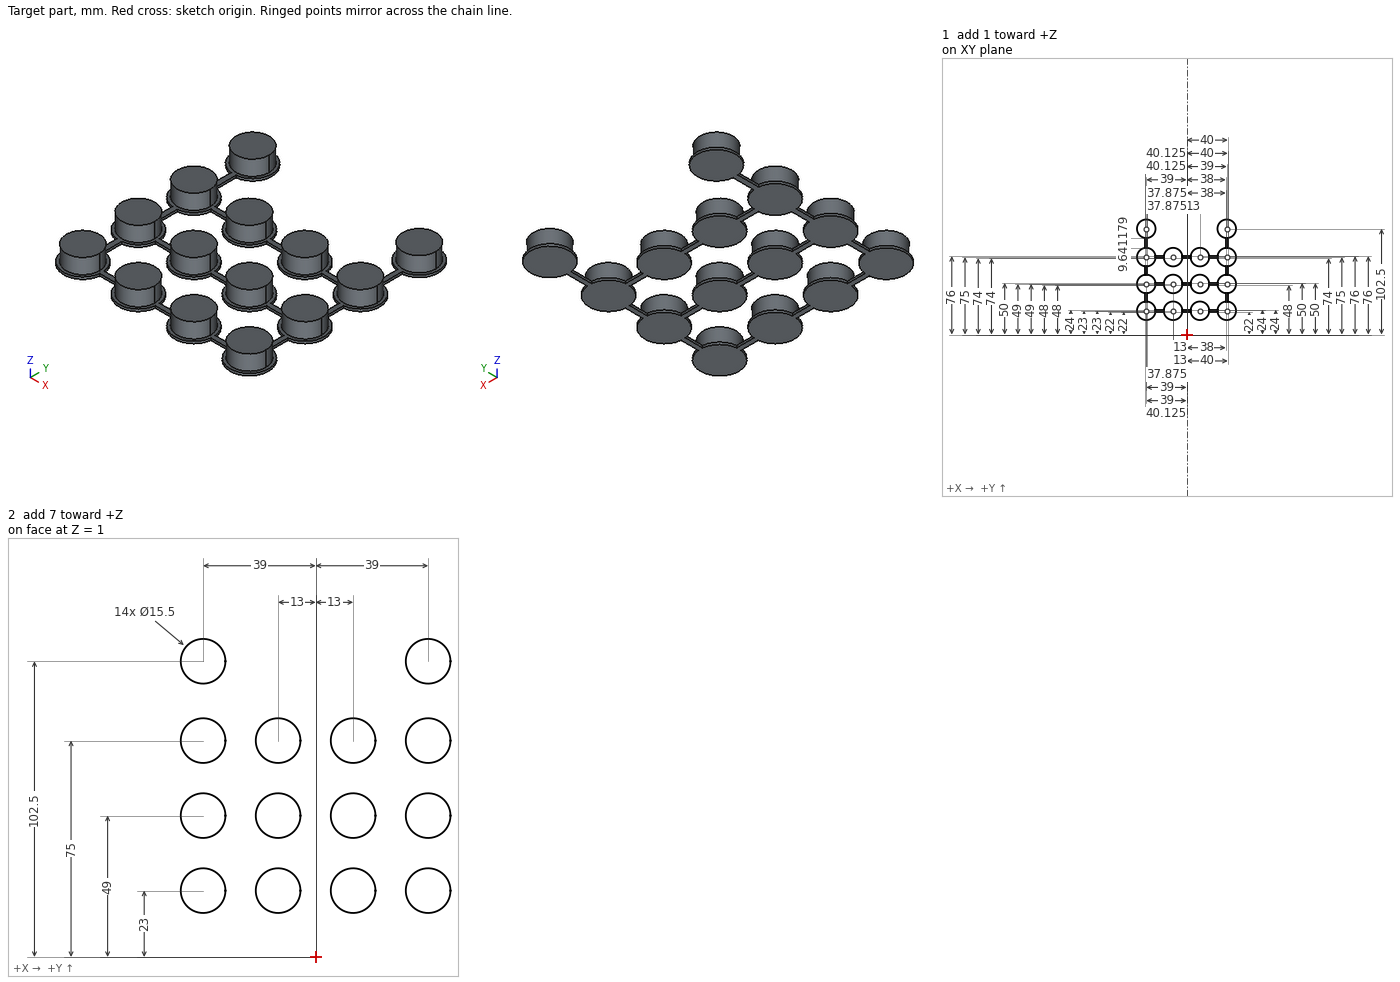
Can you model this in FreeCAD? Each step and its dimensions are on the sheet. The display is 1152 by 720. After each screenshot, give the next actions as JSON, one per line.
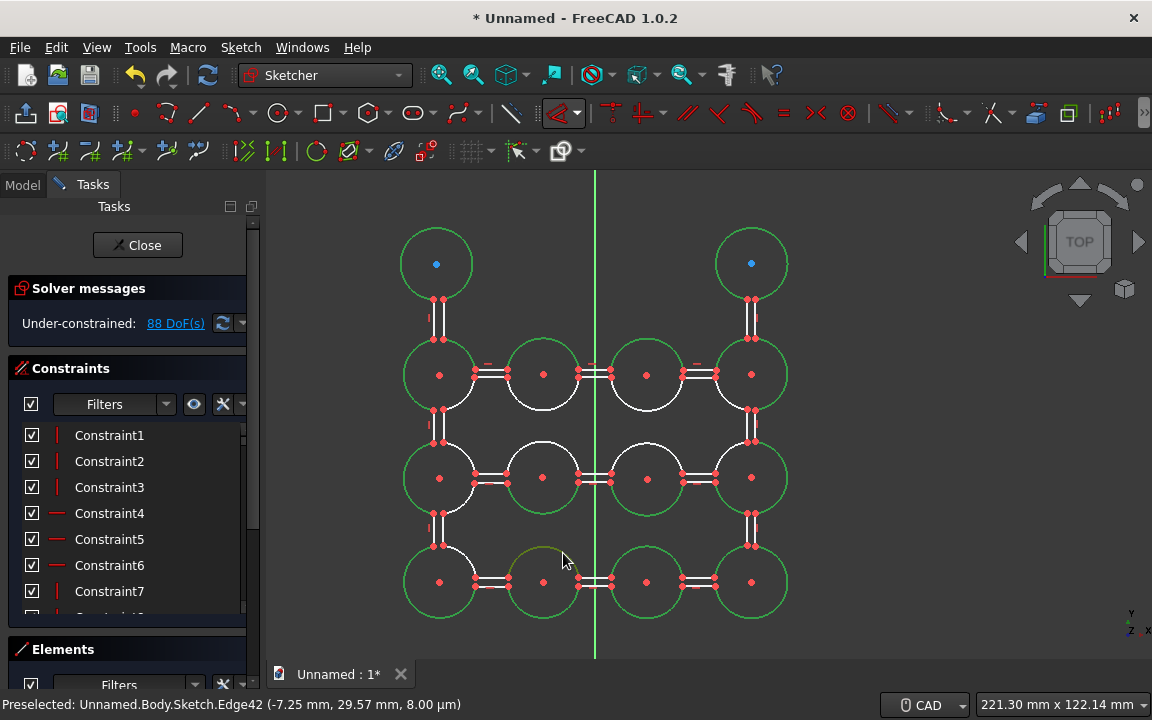
{"action": "left_click", "coordinate": [471, 564]}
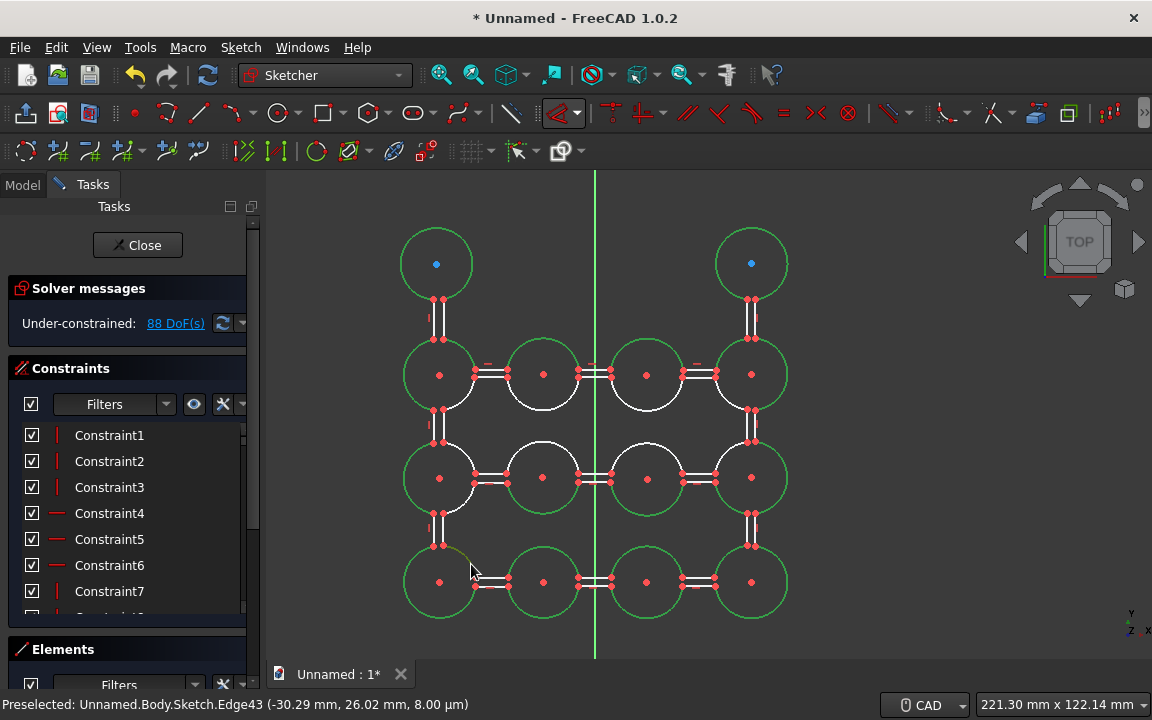
{"action": "left_click", "coordinate": [457, 509]}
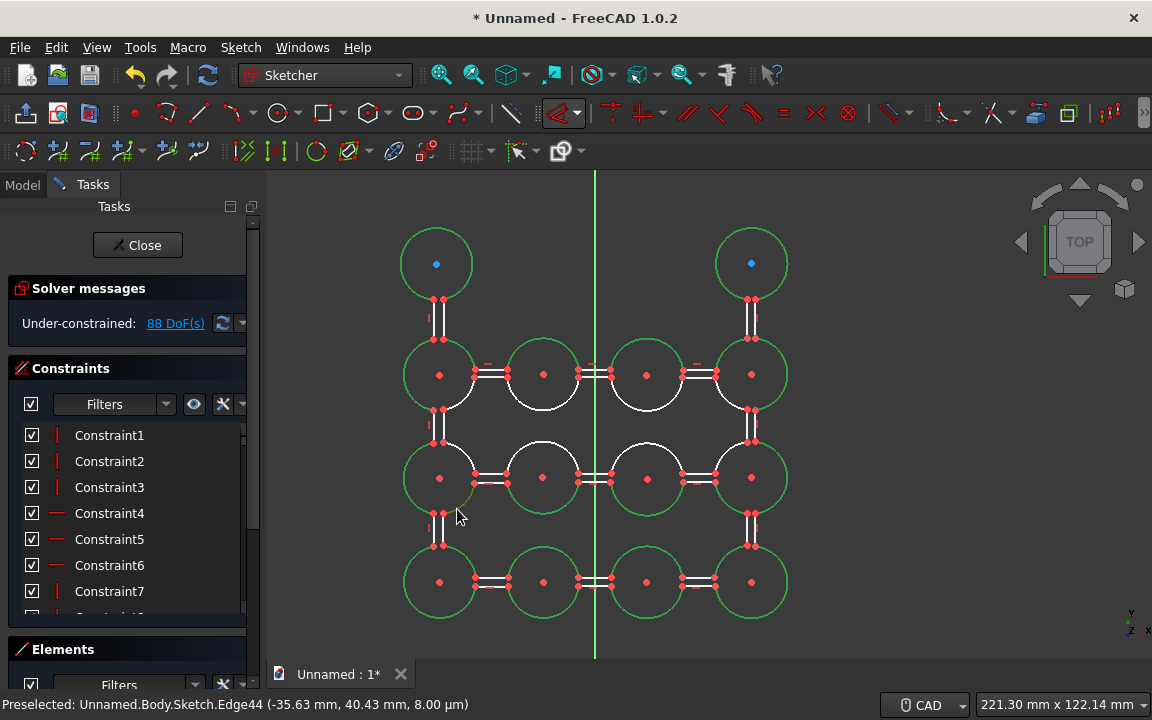
{"action": "left_click", "coordinate": [523, 404]}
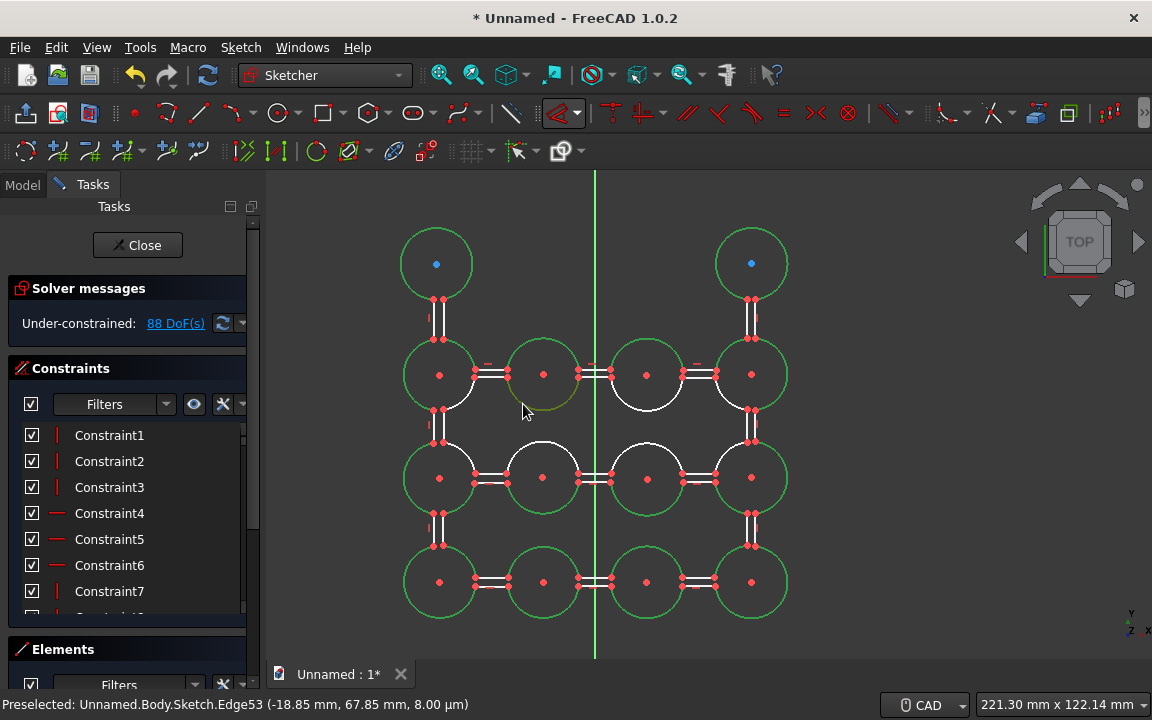
{"action": "left_click", "coordinate": [627, 405]}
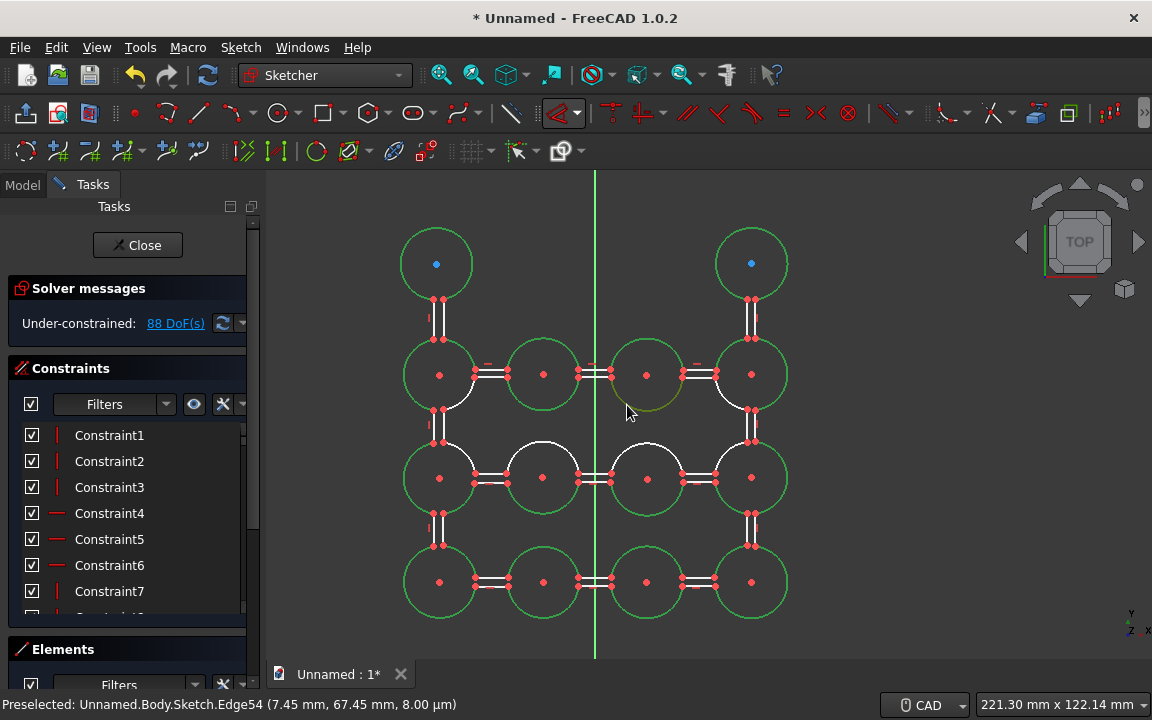
{"action": "left_click", "coordinate": [720, 392]}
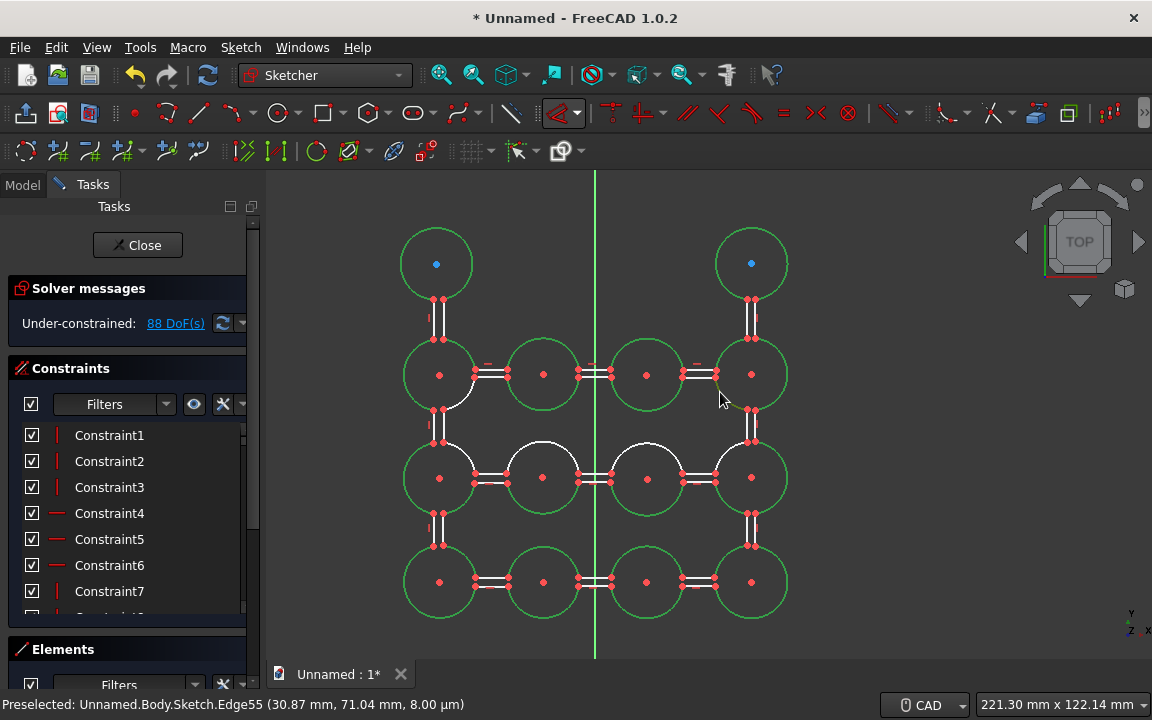
{"action": "left_click", "coordinate": [734, 446]}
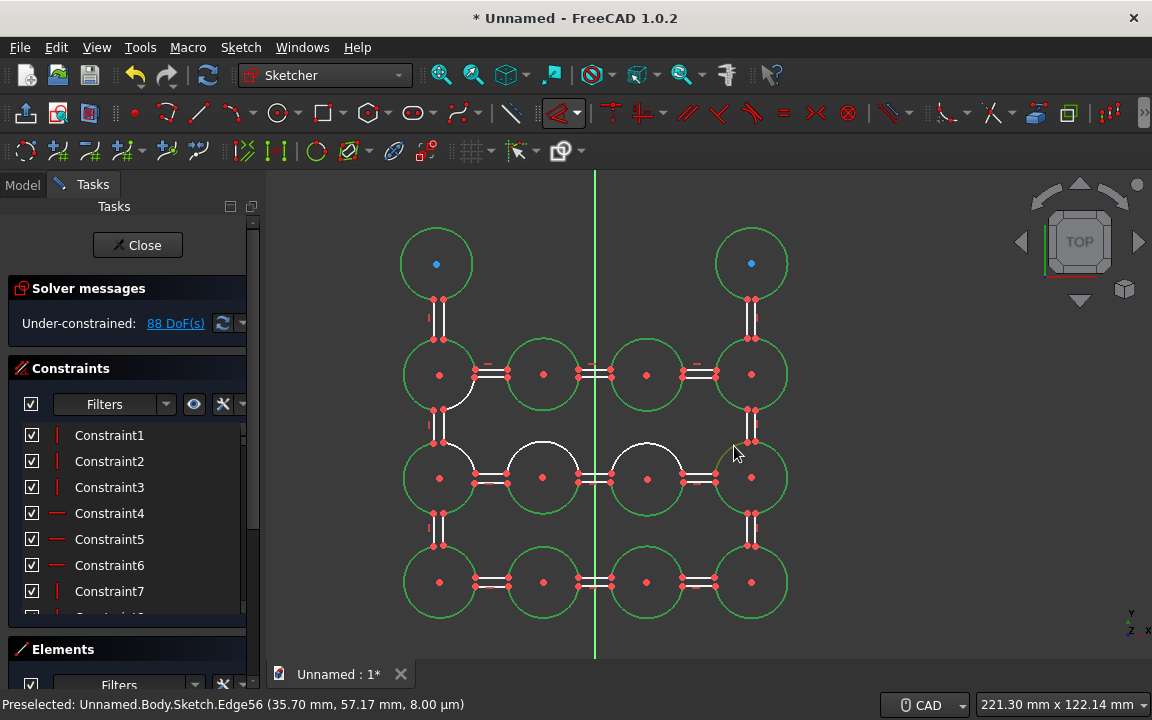
{"action": "left_click", "coordinate": [666, 449]}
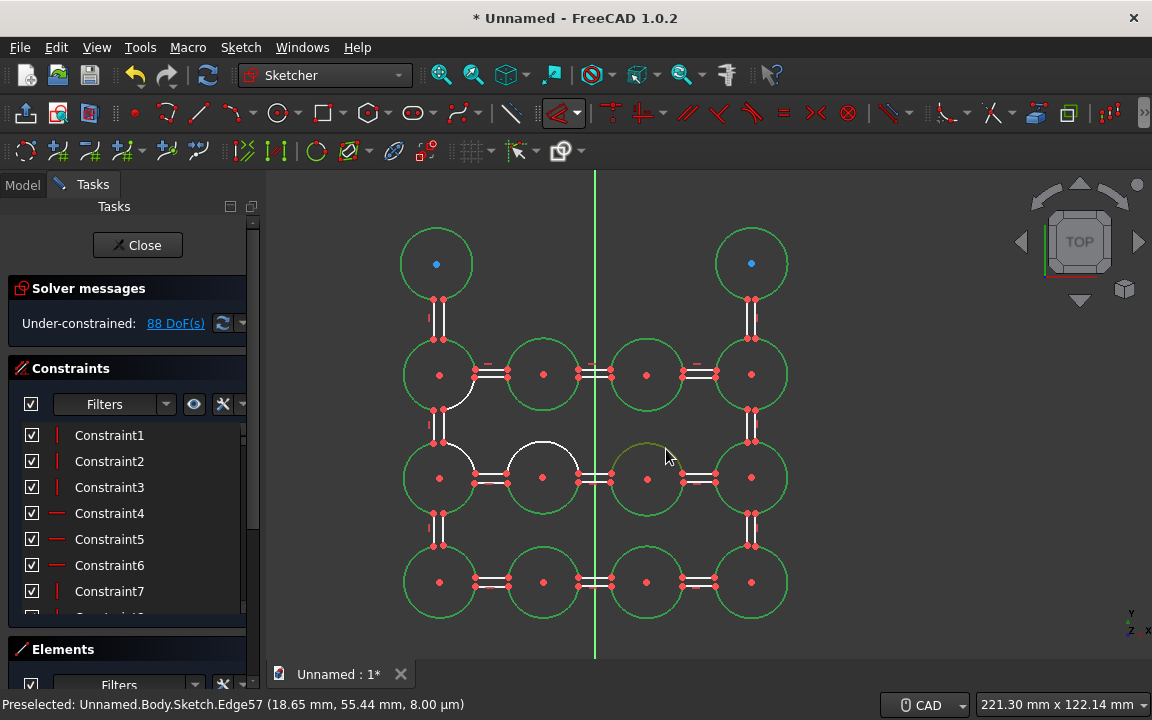
{"action": "left_click", "coordinate": [563, 448]}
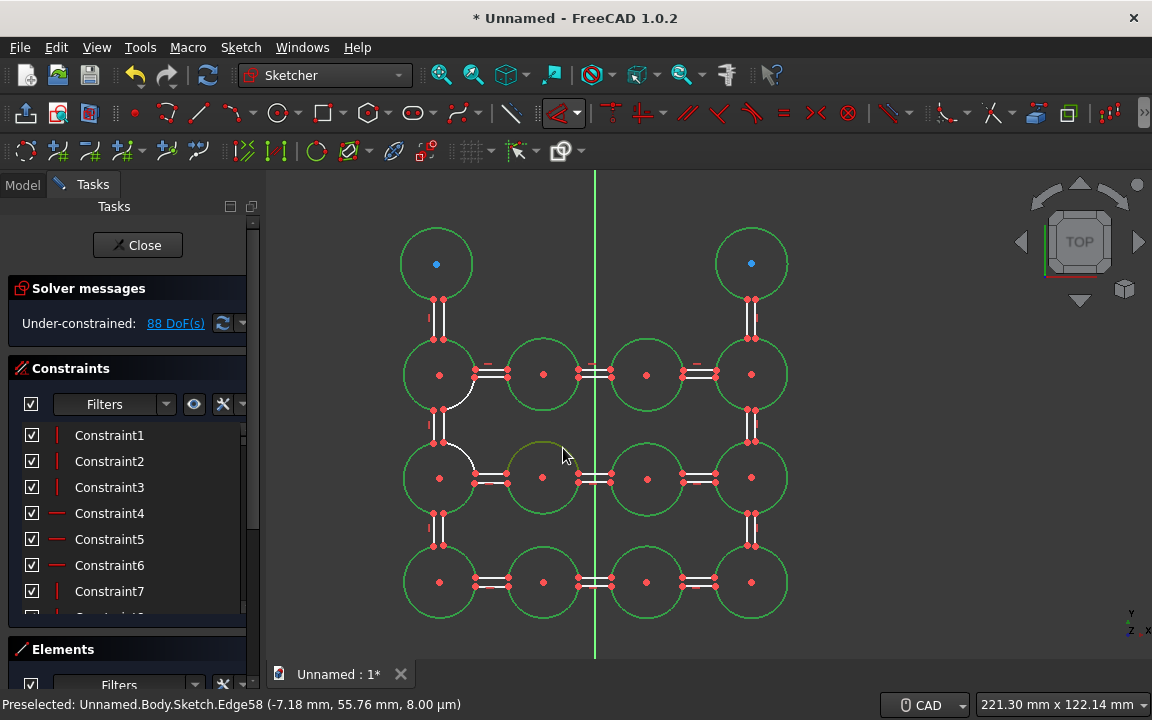
{"action": "left_click", "coordinate": [471, 460]}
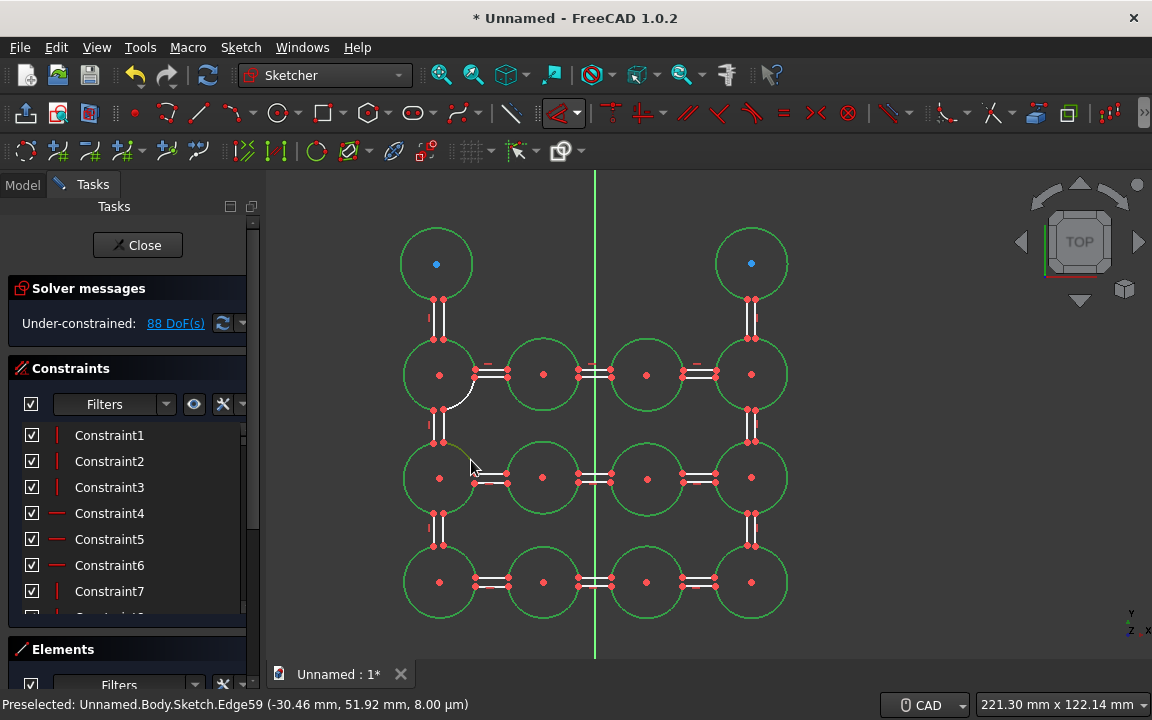
{"action": "left_click", "coordinate": [457, 405]}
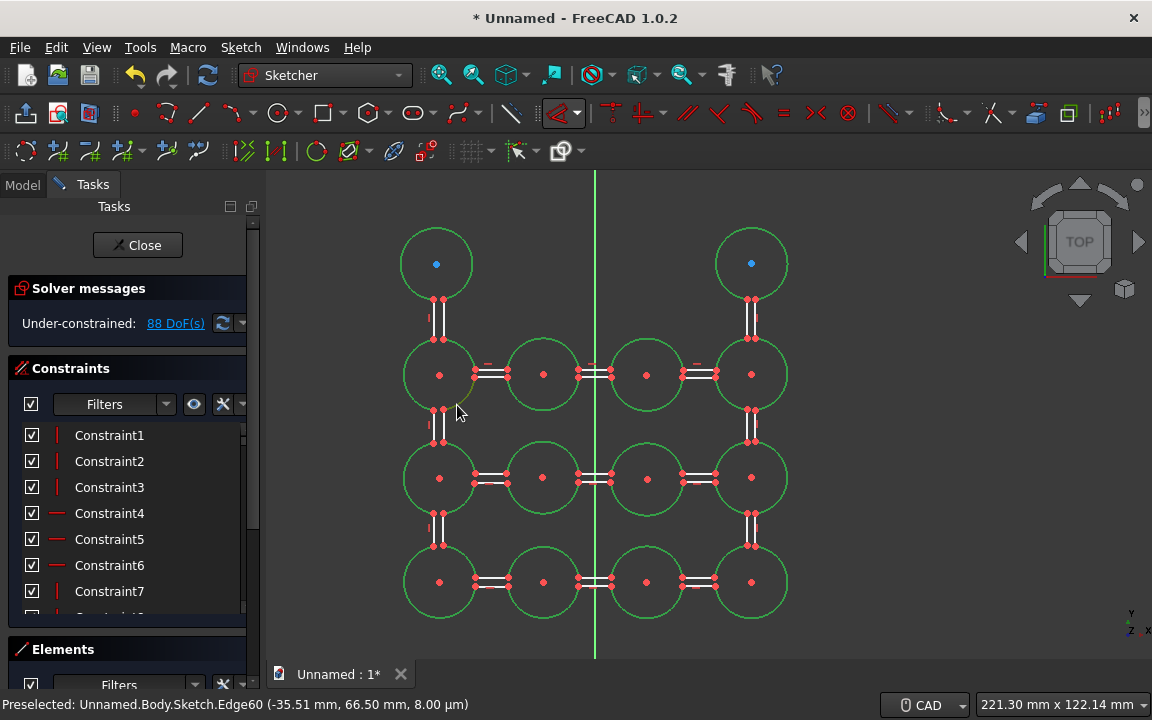
{"action": "left_click", "coordinate": [784, 114]}